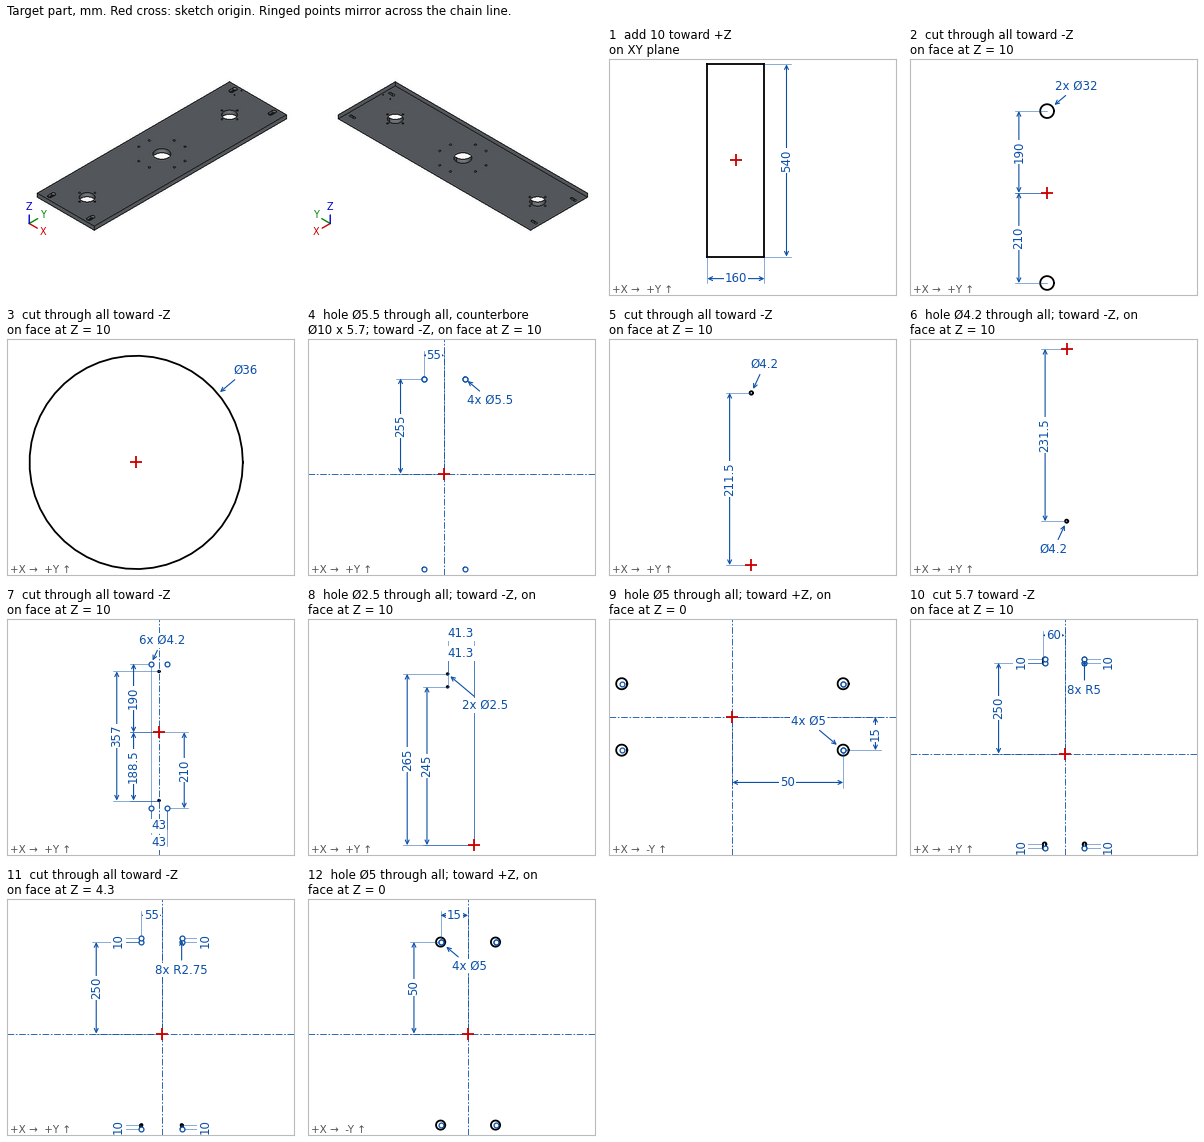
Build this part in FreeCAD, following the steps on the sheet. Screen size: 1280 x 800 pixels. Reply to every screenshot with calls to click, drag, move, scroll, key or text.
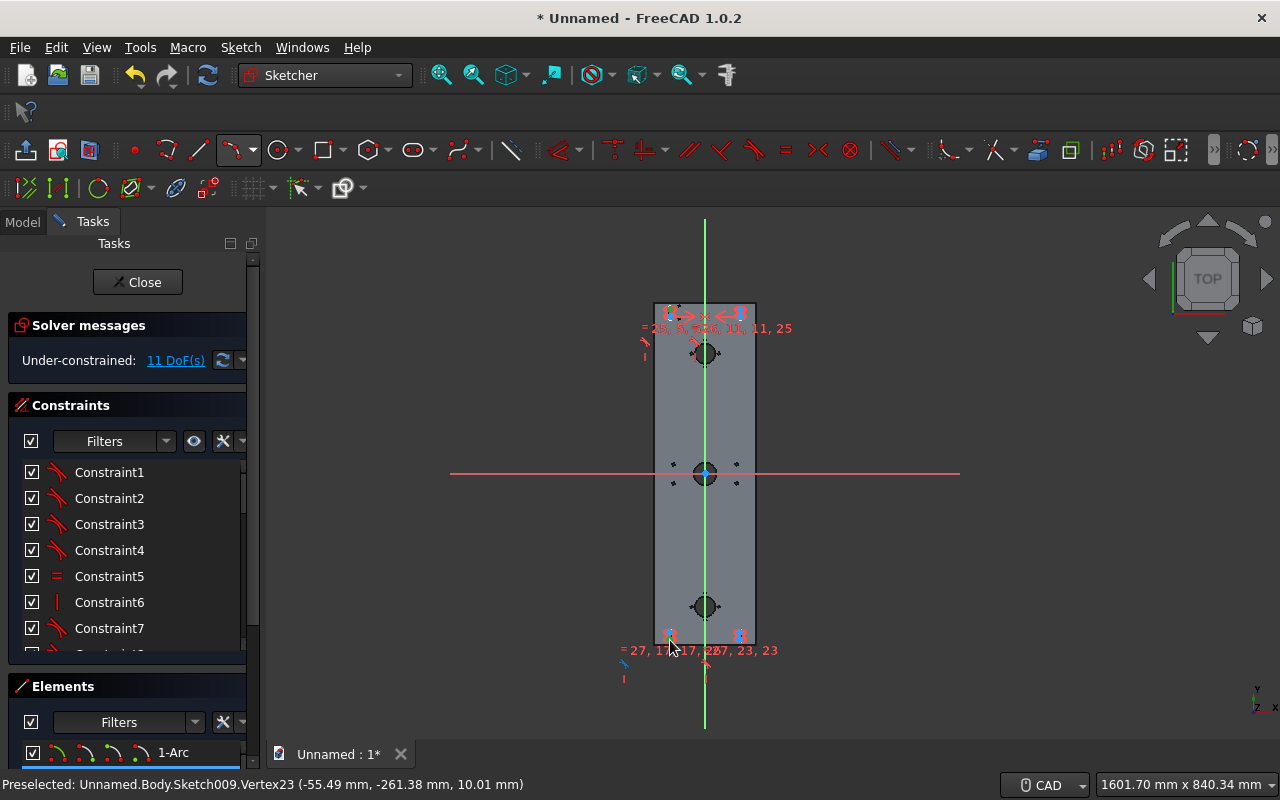
click(470, 474)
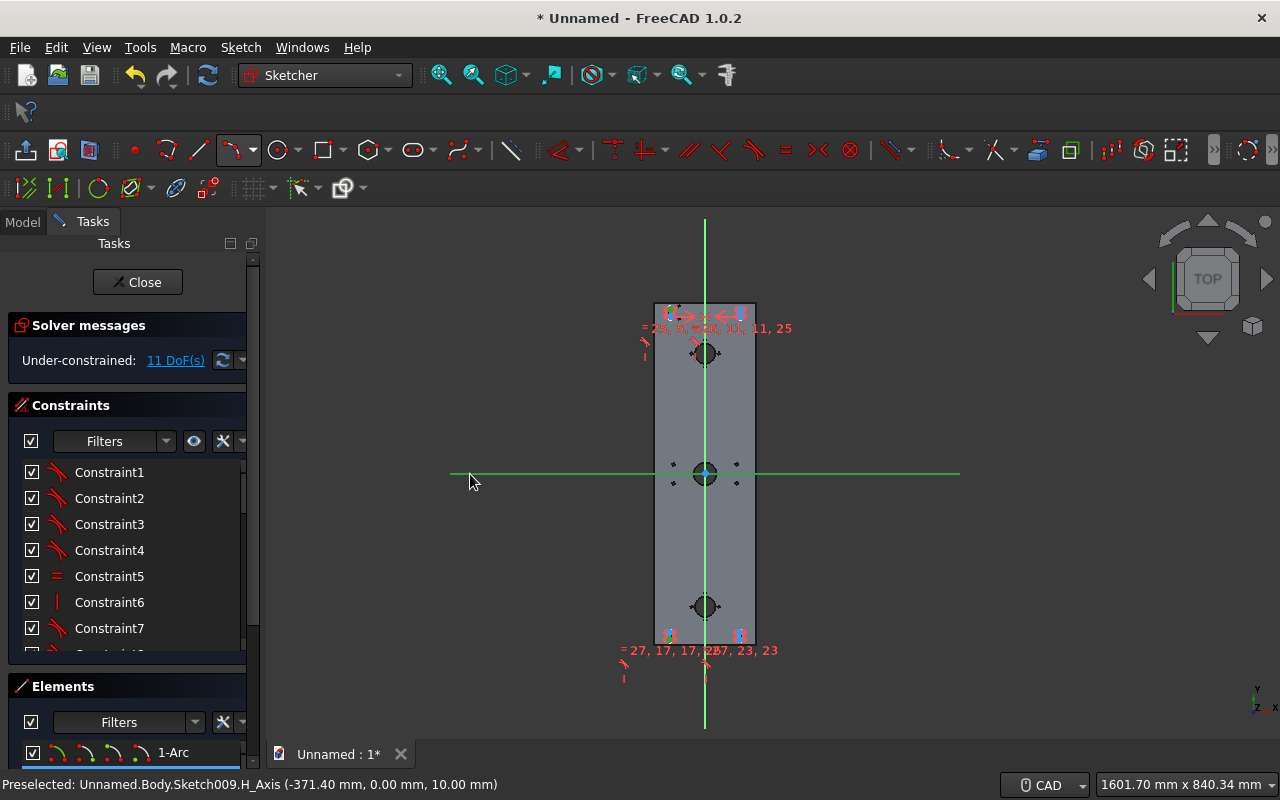
click(818, 150)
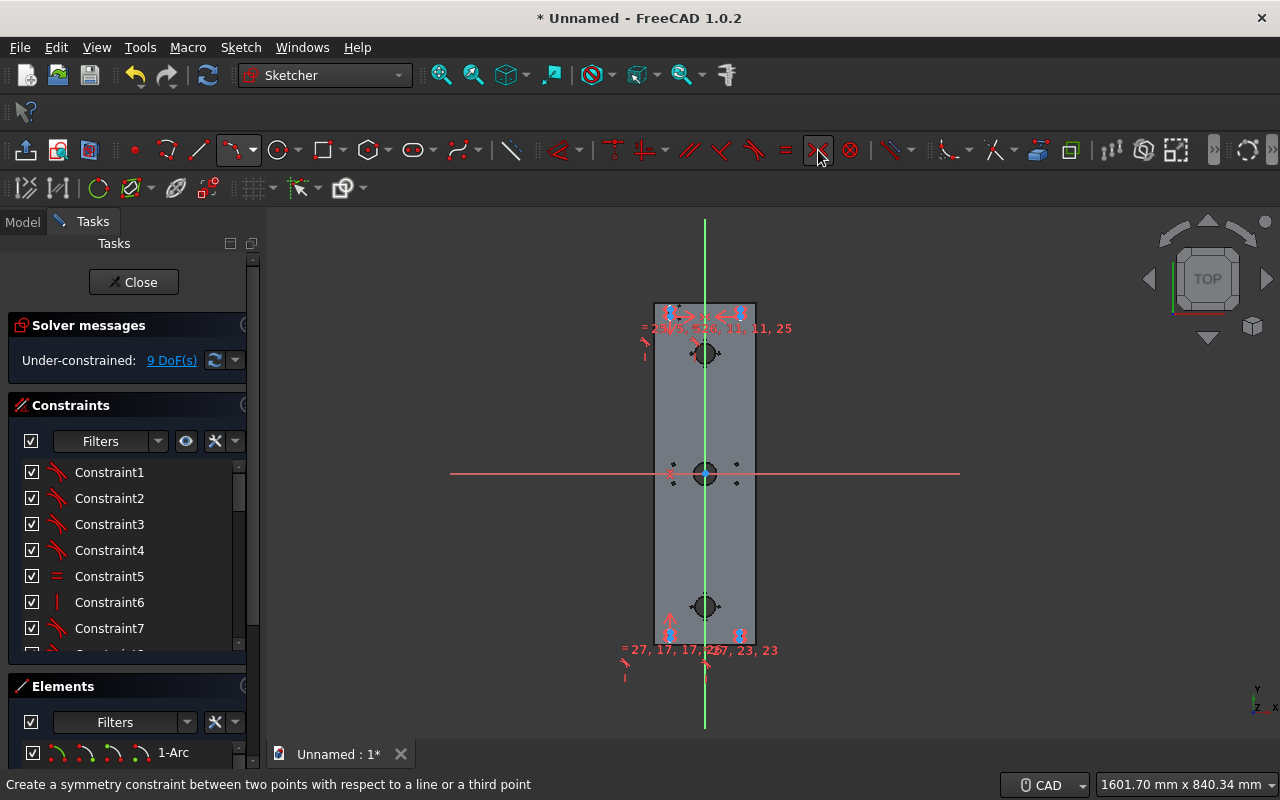
scroll(740, 310, up, 7)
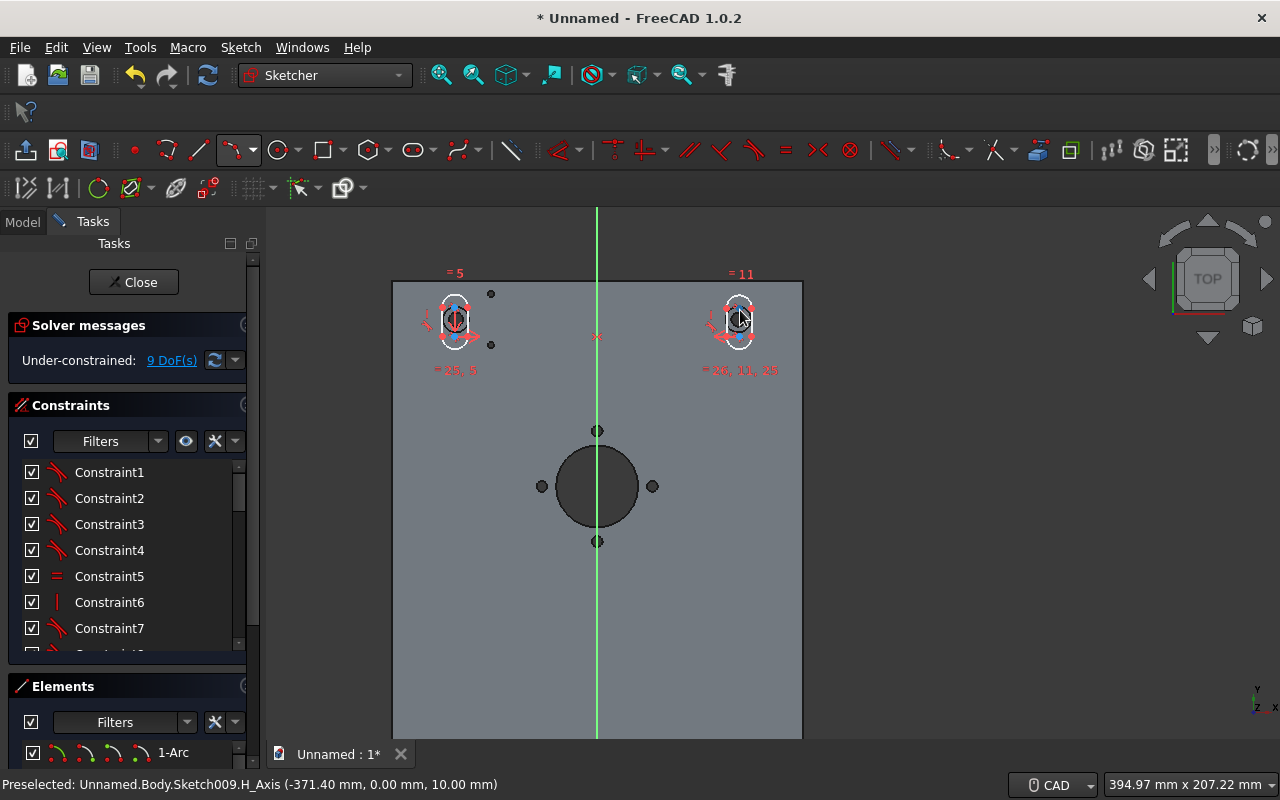
click(739, 308)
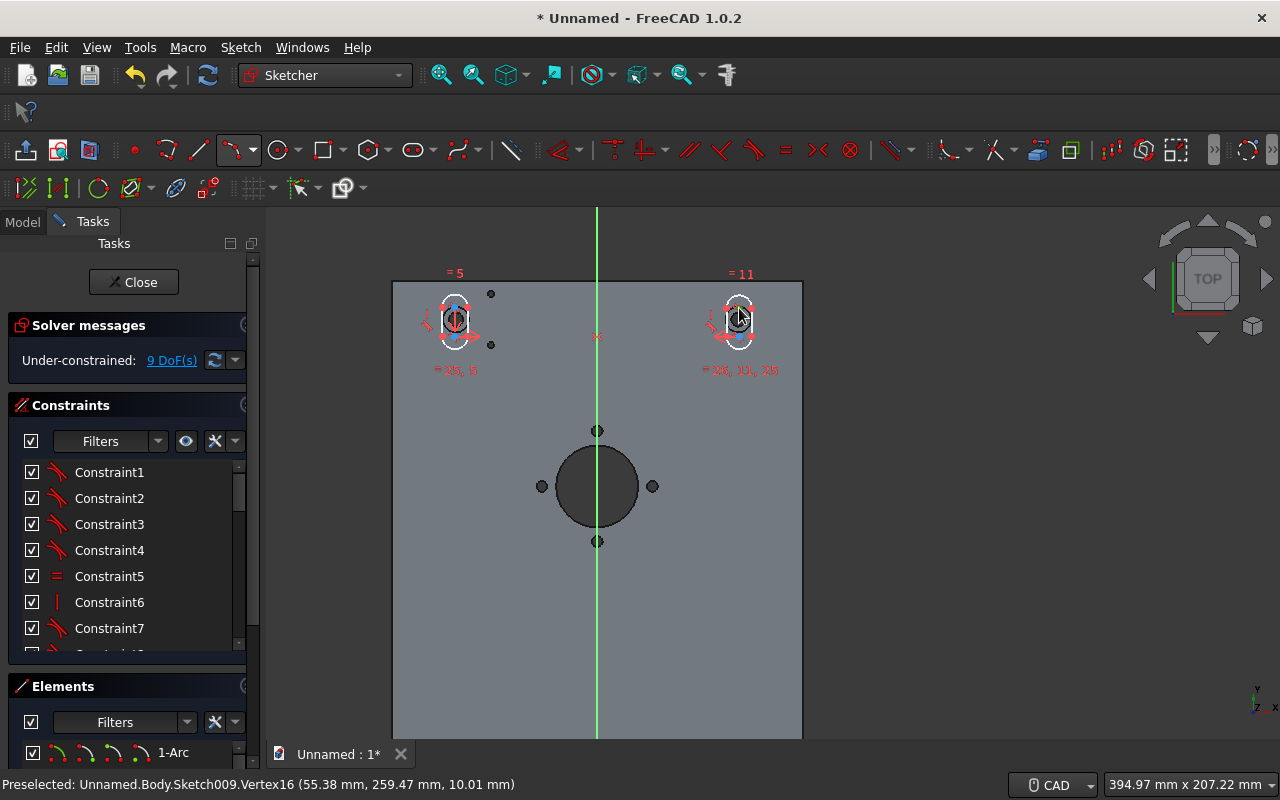
scroll(740, 309, down, 7)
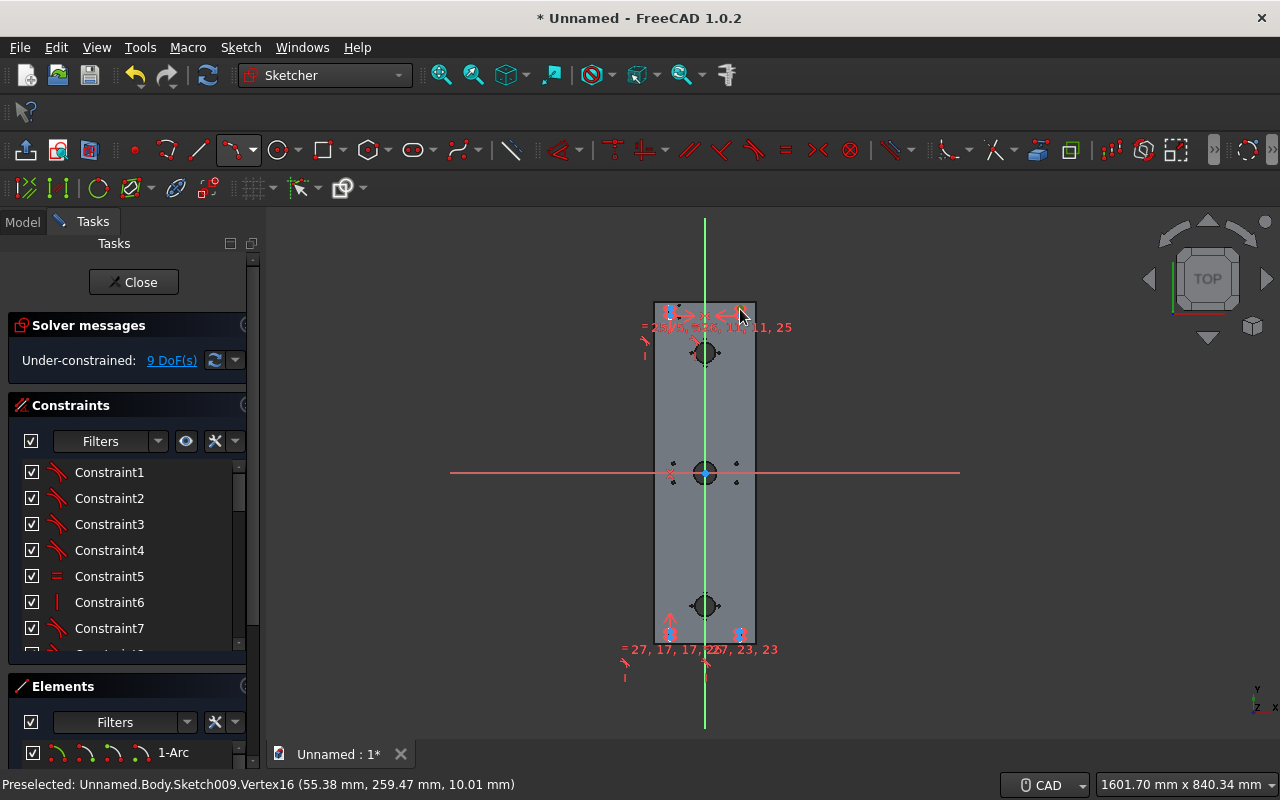
scroll(740, 638, up, 7)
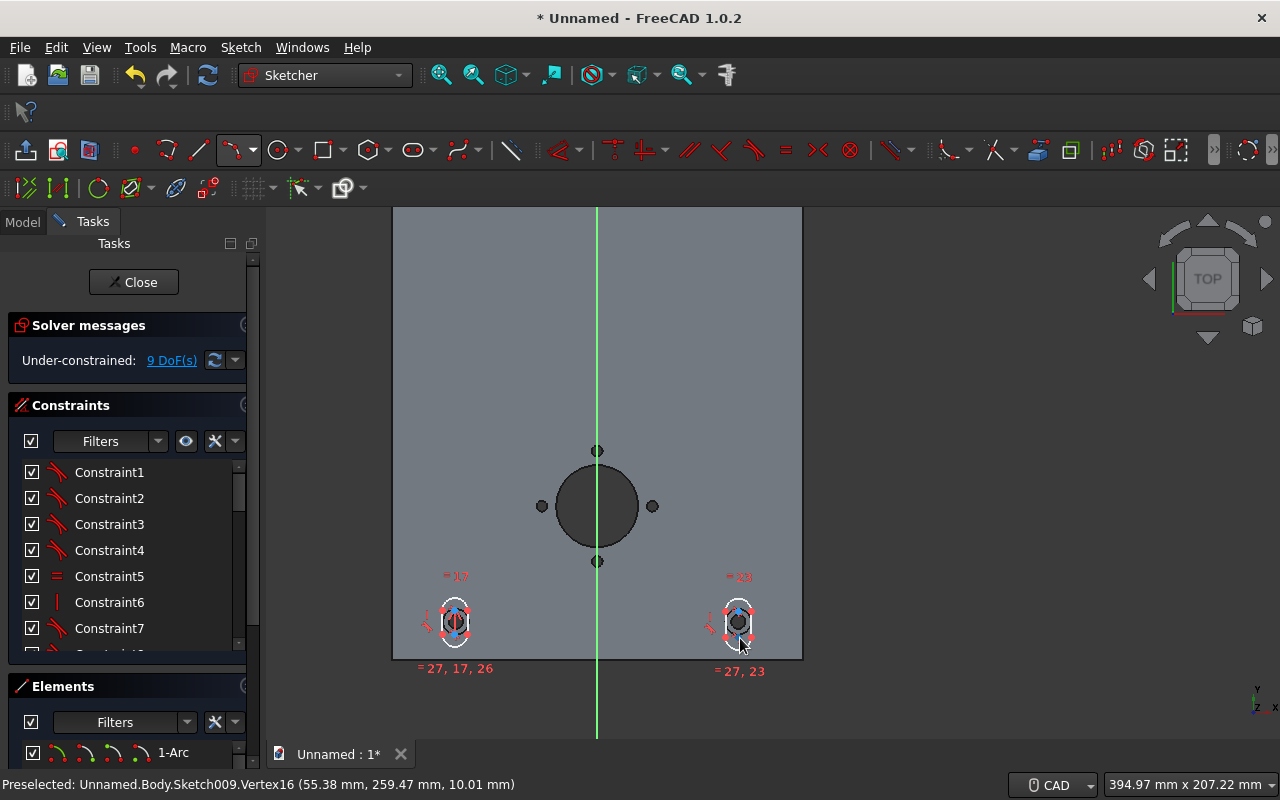
click(738, 637)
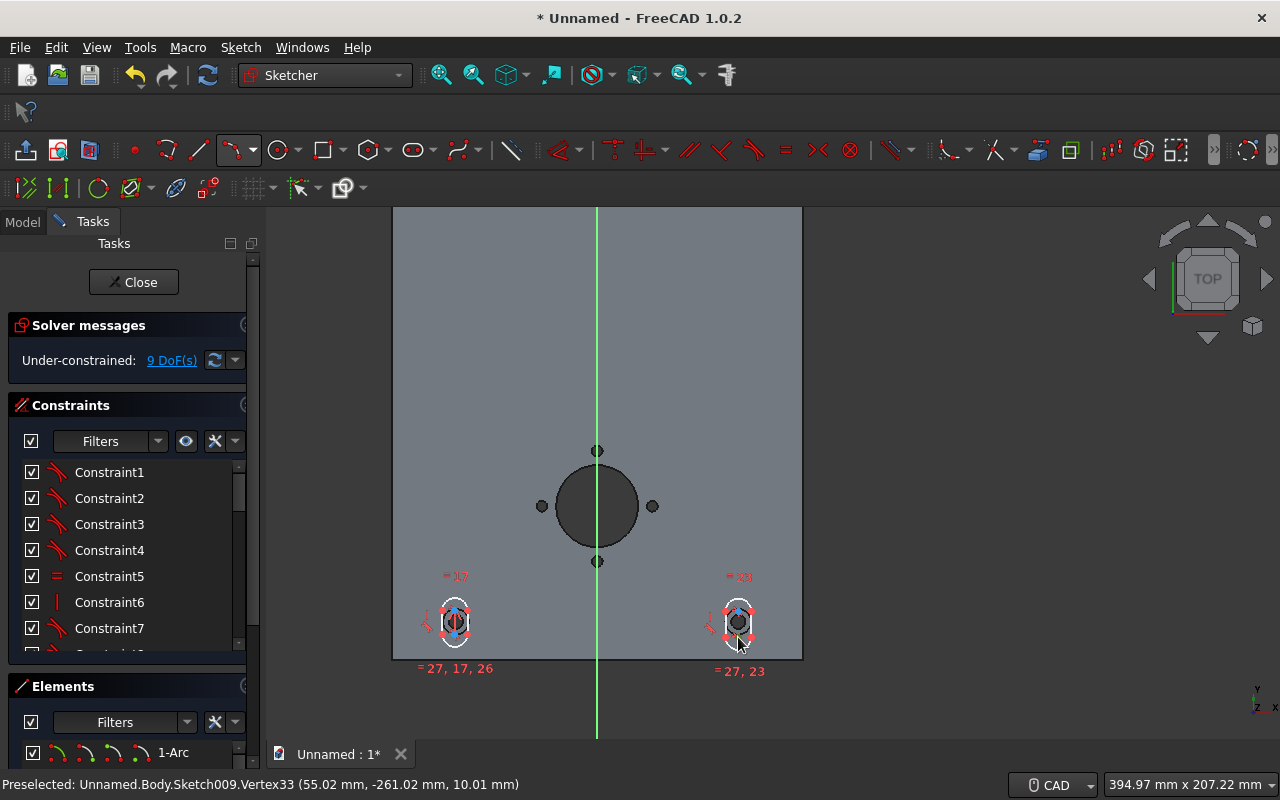
scroll(740, 639, down, 7)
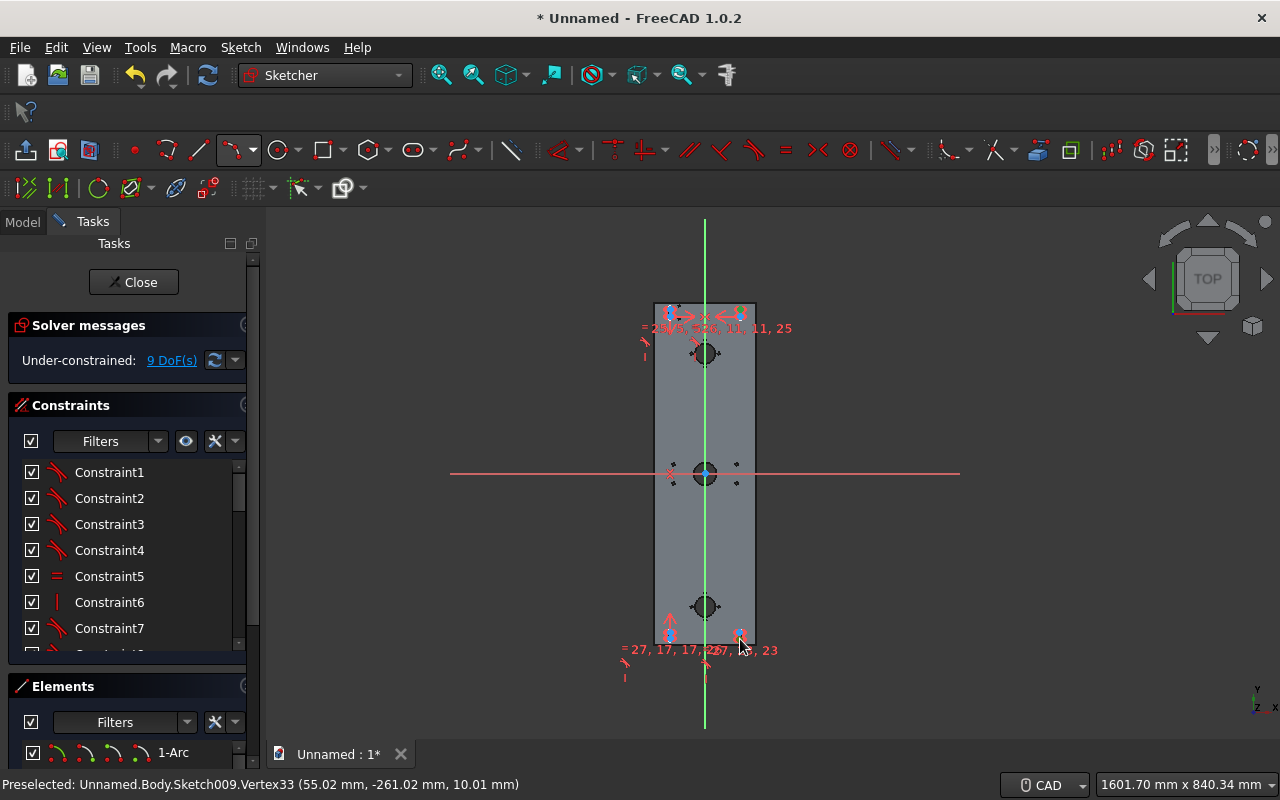
click(470, 474)